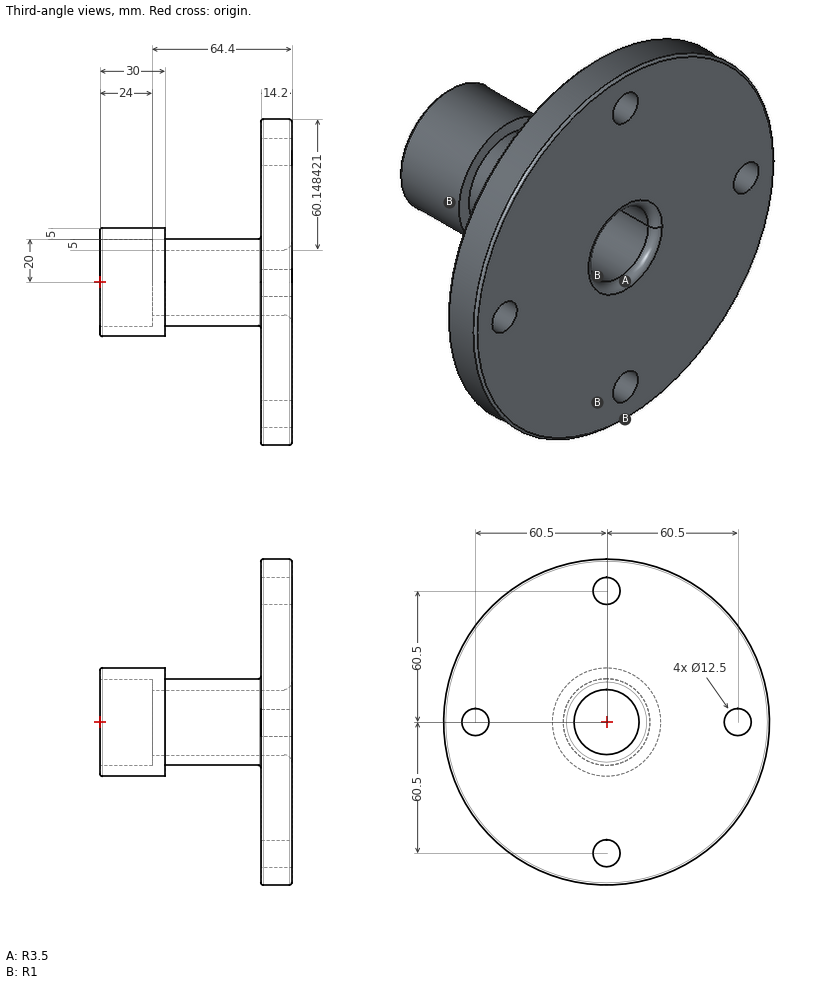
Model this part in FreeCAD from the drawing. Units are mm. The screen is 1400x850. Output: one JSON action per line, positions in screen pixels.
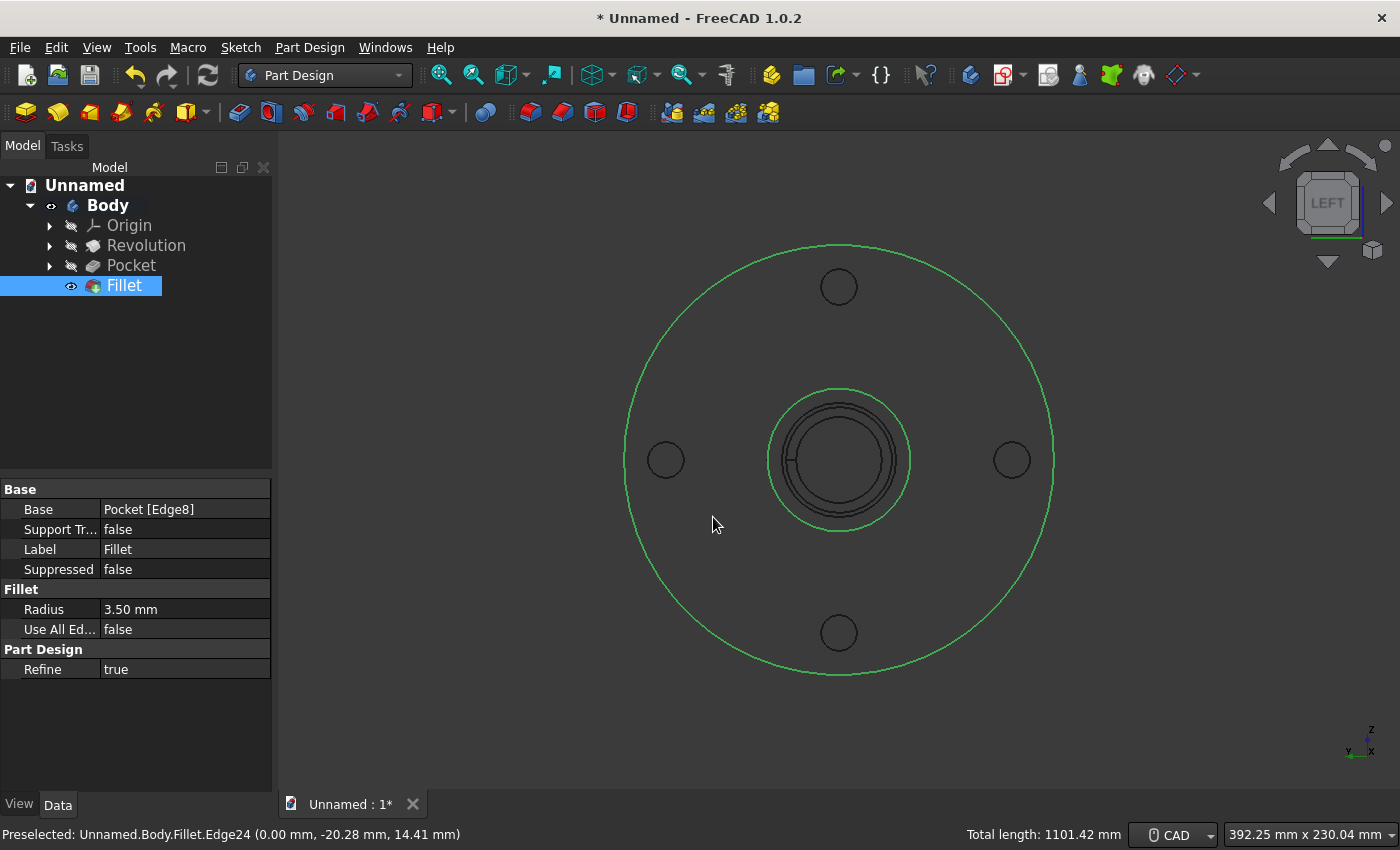
{"action": "key", "text": "0"}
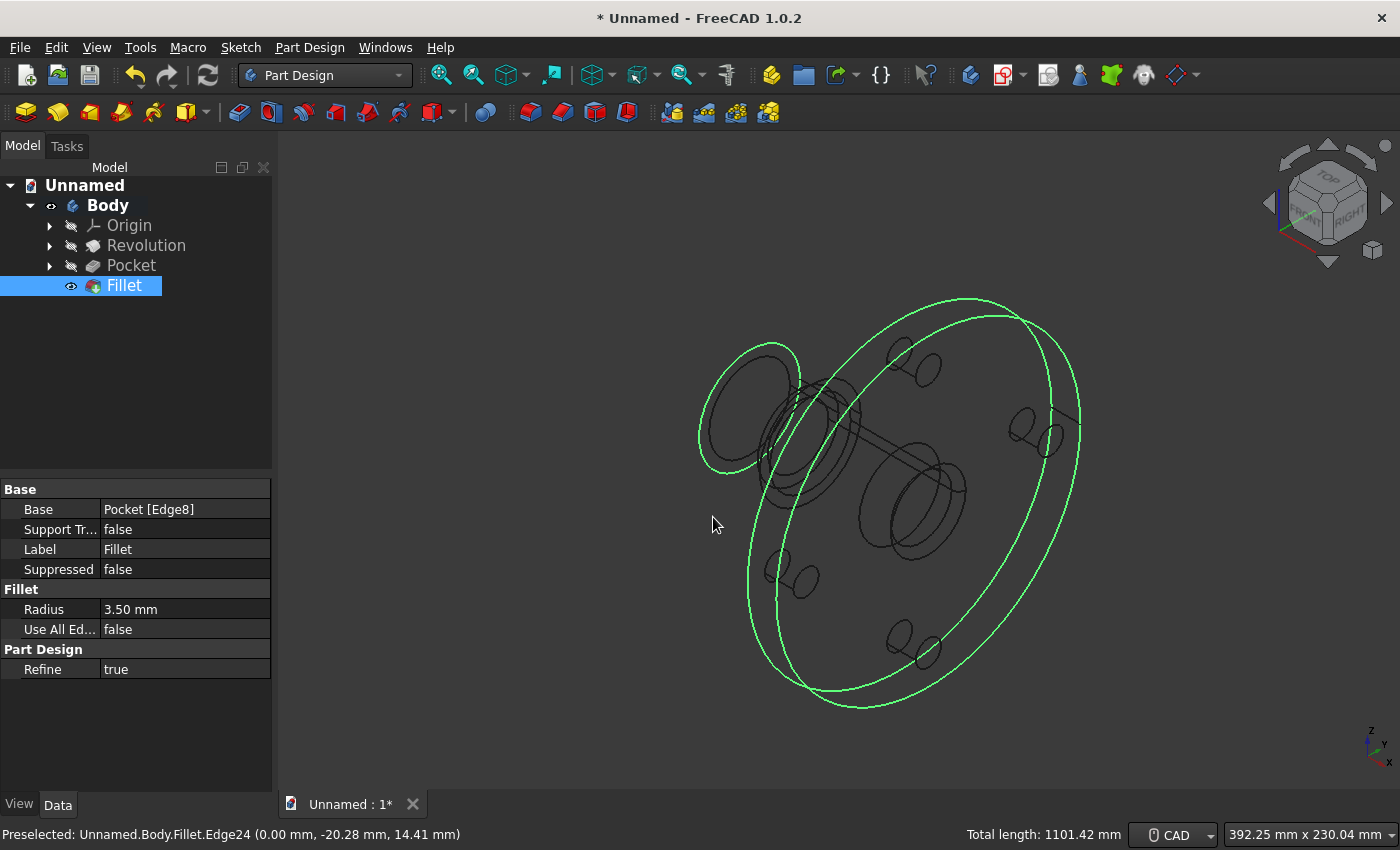
{"action": "left_click", "coordinate": [859, 517], "text": "ctrl"}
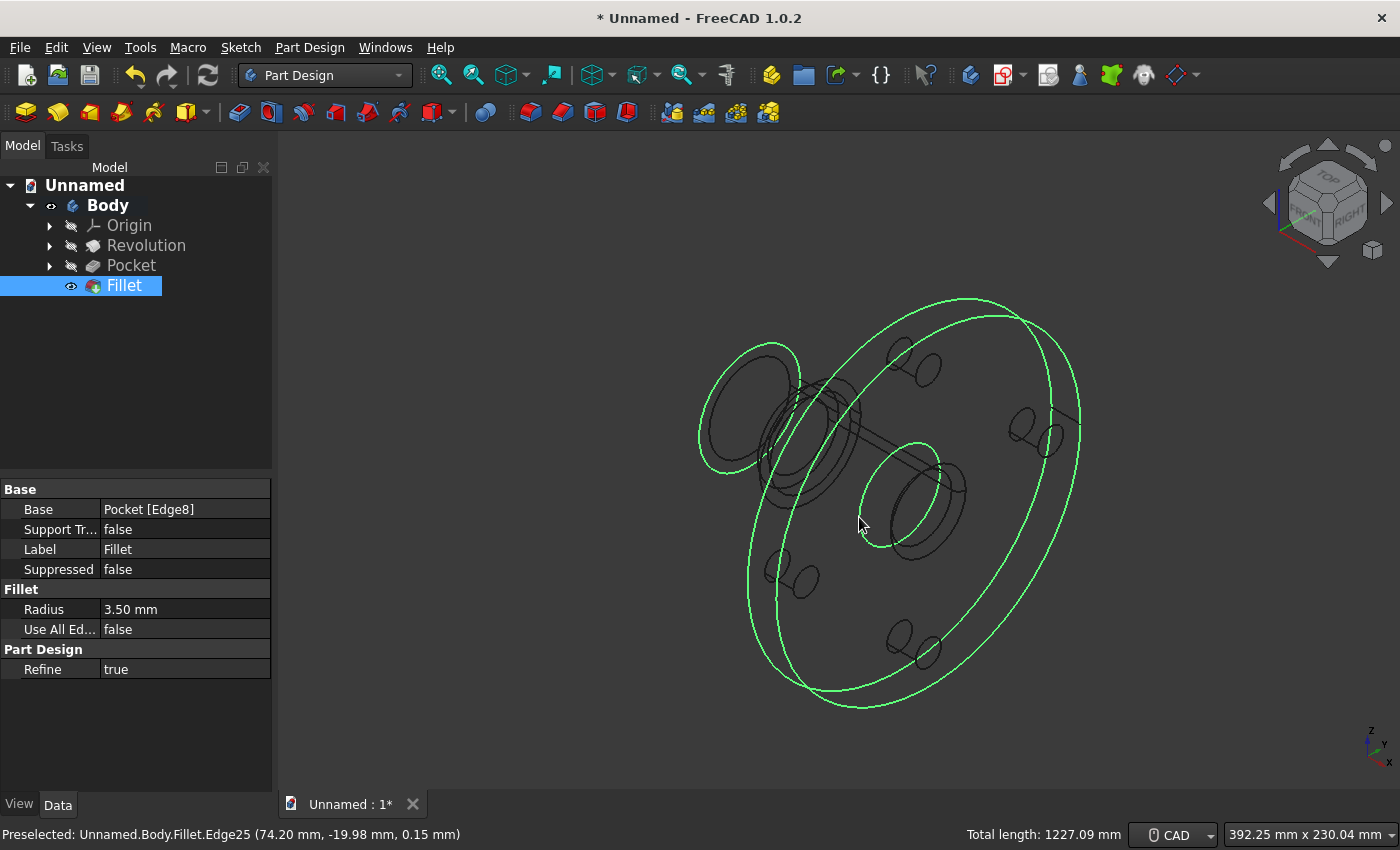
{"action": "key", "text": "v 1"}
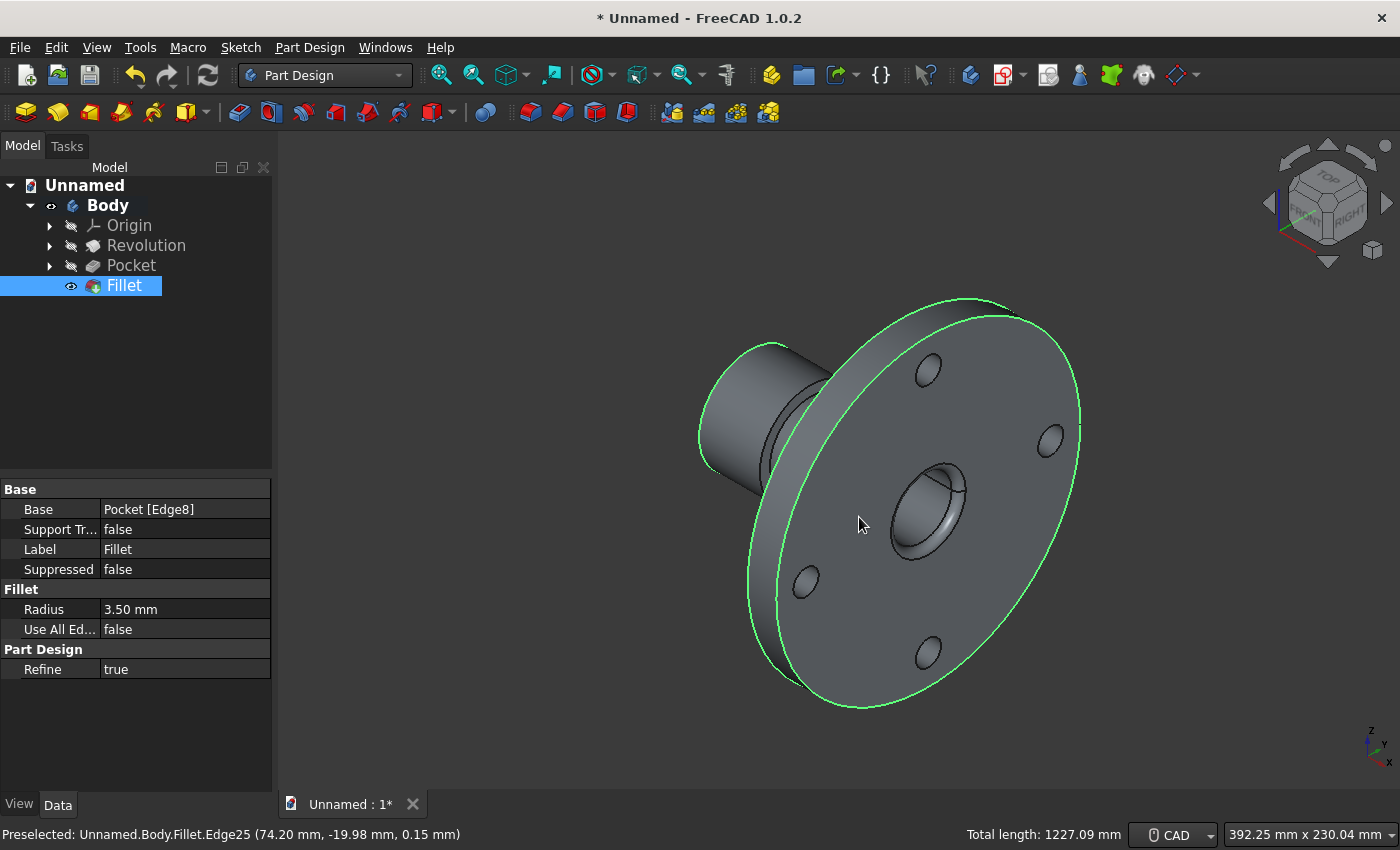
{"action": "left_click", "coordinate": [532, 112]}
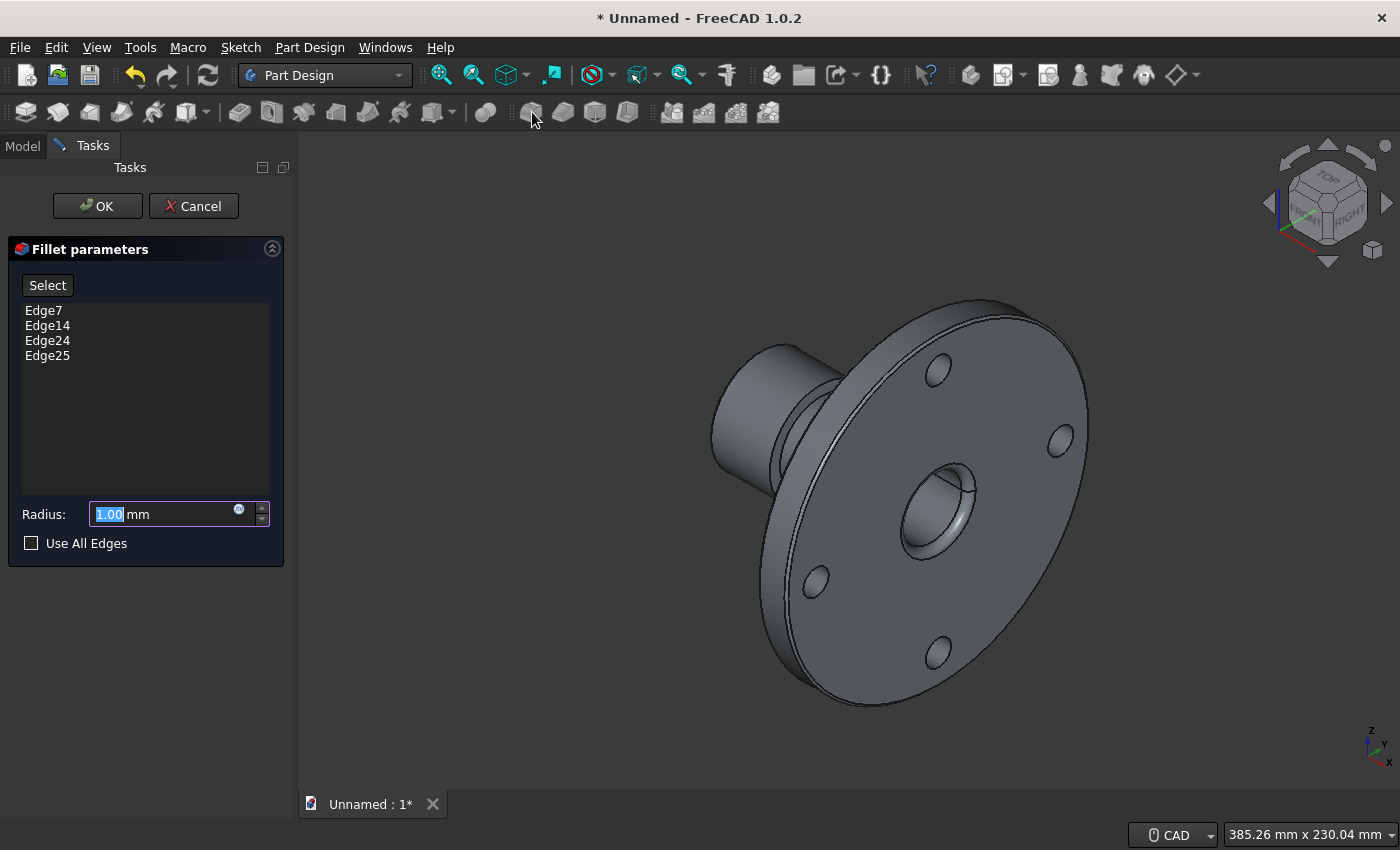
{"action": "type", "text": "1"}
{"action": "key", "text": "Tab"}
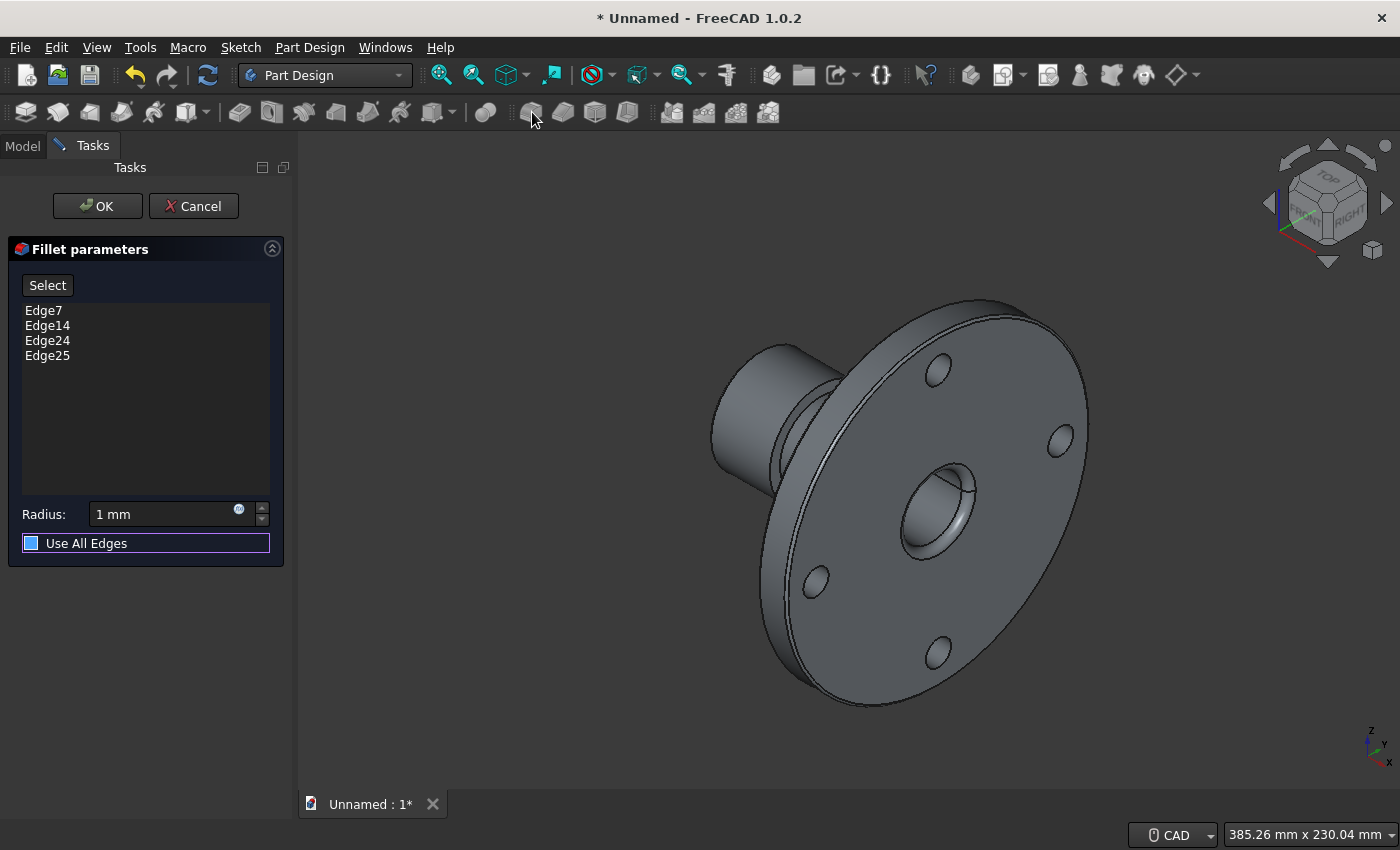
{"action": "left_click", "coordinate": [98, 206]}